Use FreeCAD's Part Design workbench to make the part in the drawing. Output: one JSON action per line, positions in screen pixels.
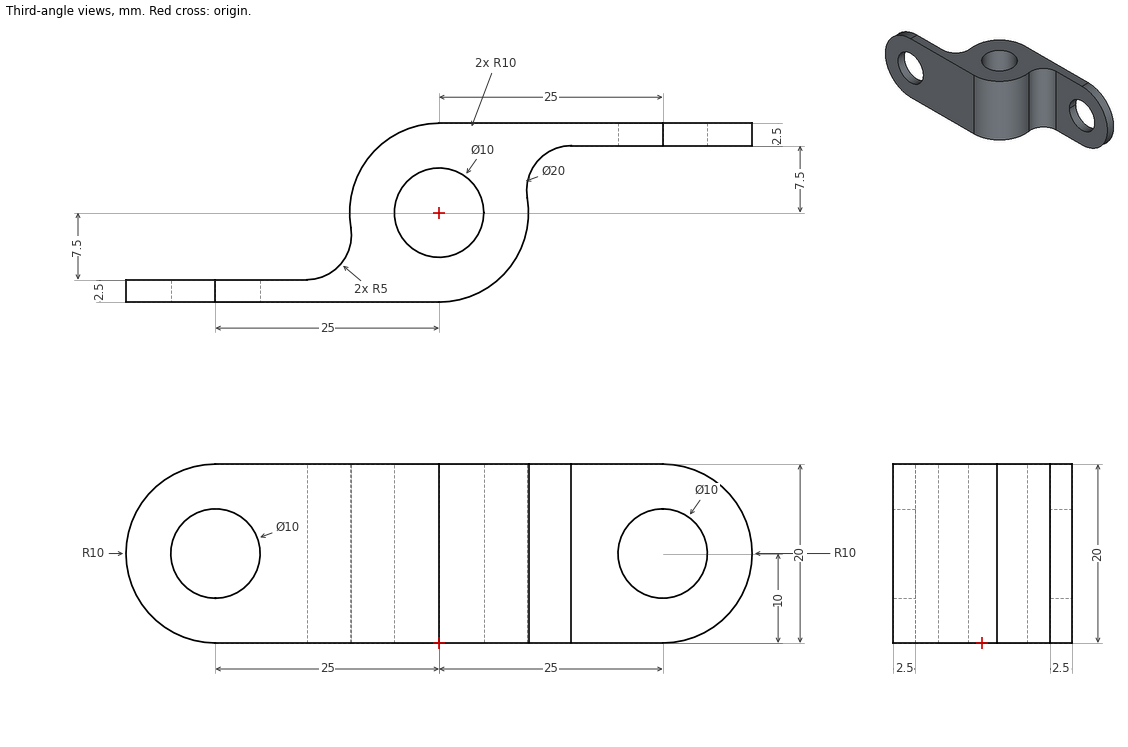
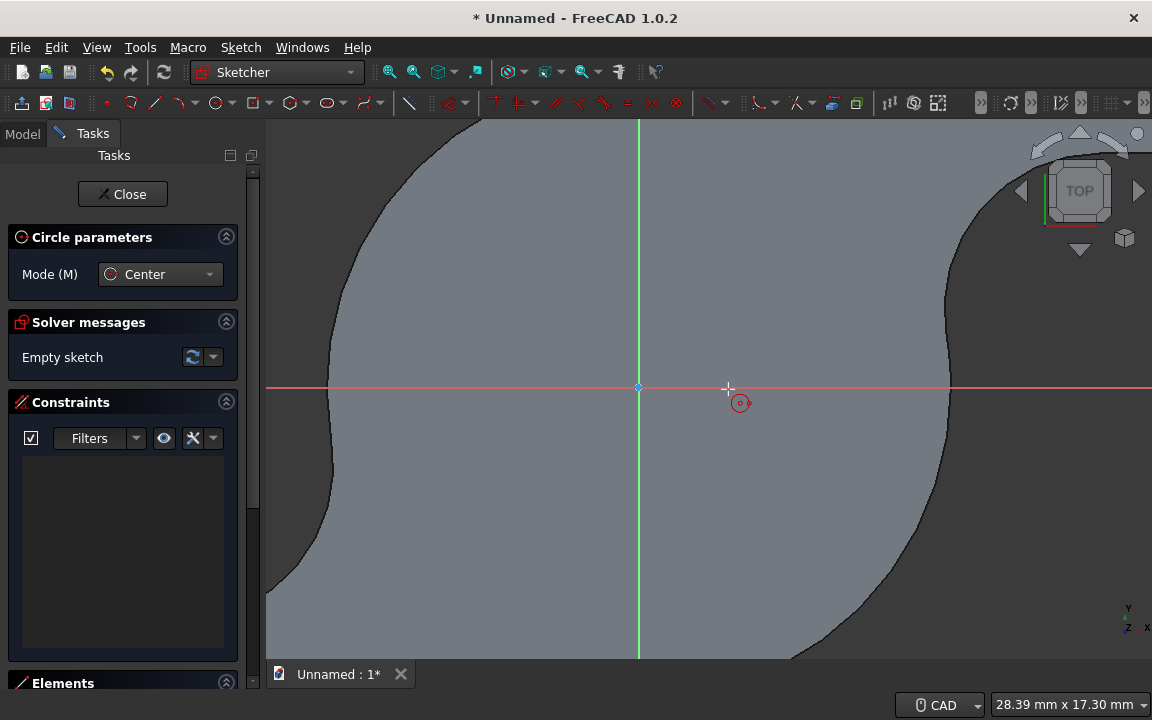
{"action": "left_click", "coordinate": [639, 388]}
{"action": "left_click", "coordinate": [749, 277]}
{"action": "key", "text": "Escape"}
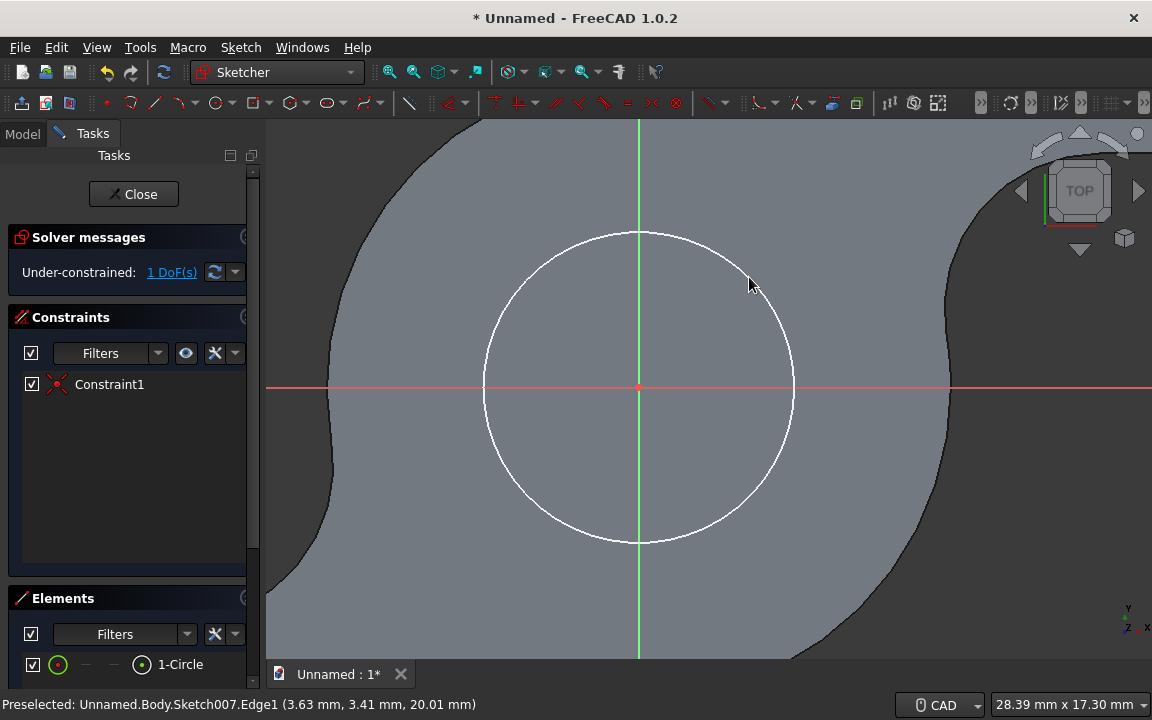
{"action": "left_click", "coordinate": [448, 104]}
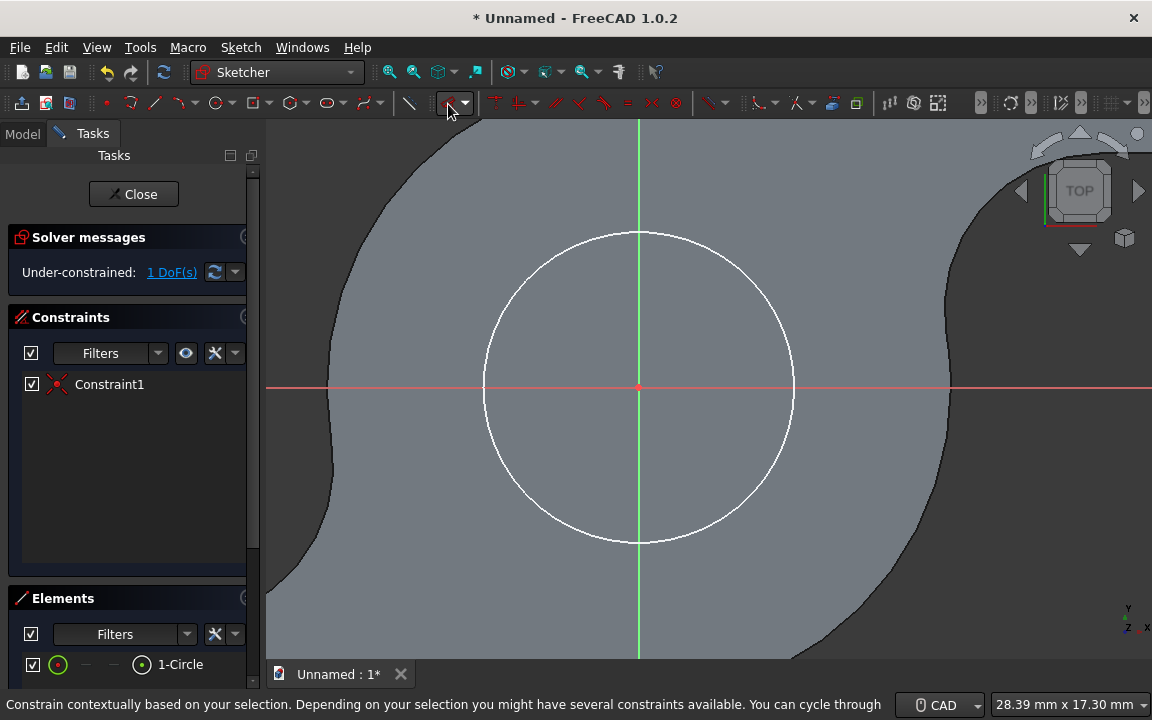
{"action": "left_click", "coordinate": [748, 277]}
{"action": "left_click", "coordinate": [770, 254]}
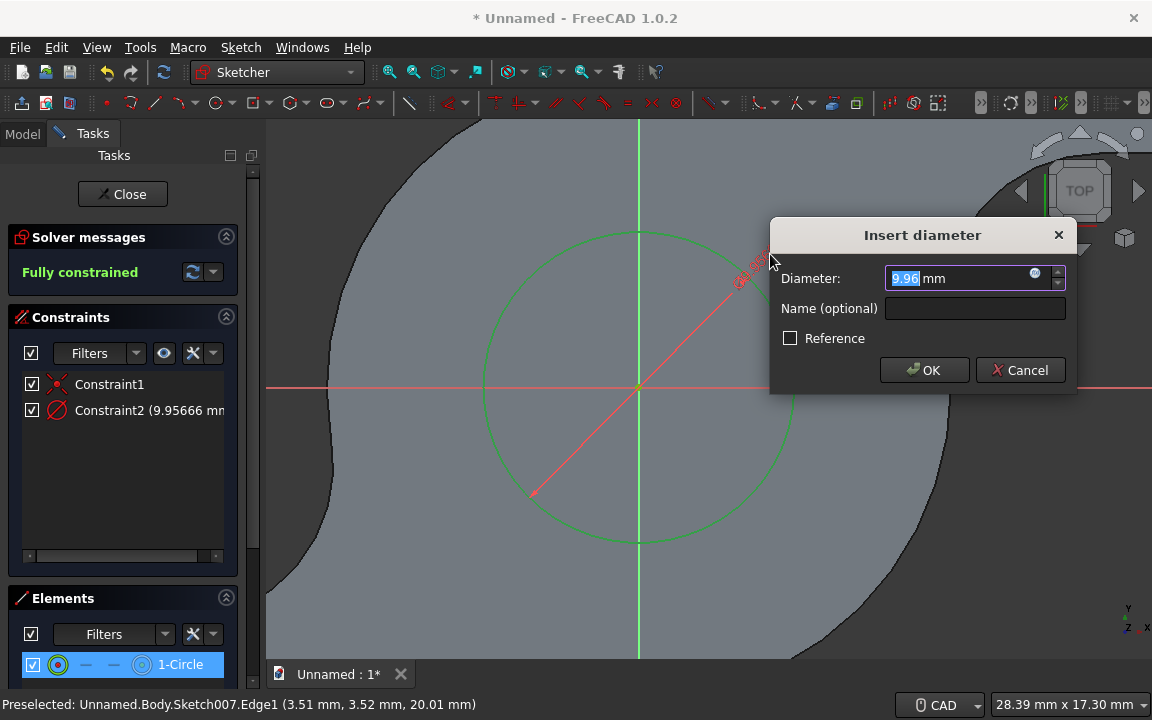
{"action": "type", "text": "10"}
{"action": "key", "text": "Return"}
{"action": "key", "text": "Escape"}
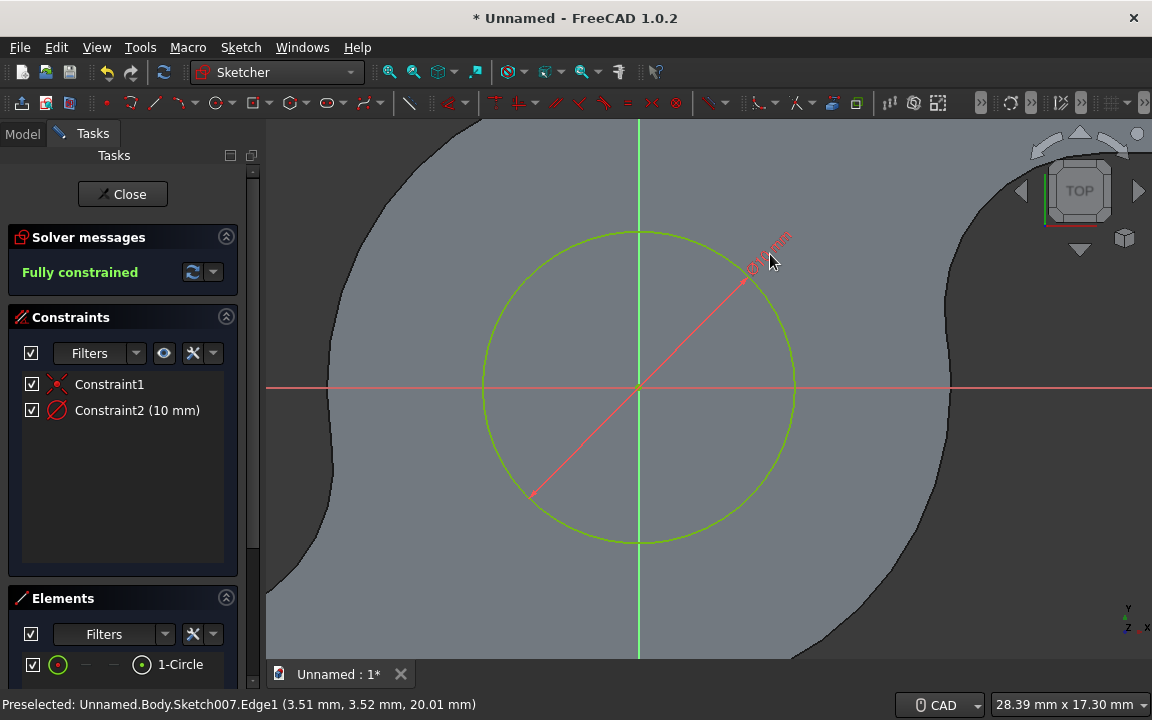
{"action": "left_click", "coordinate": [123, 194]}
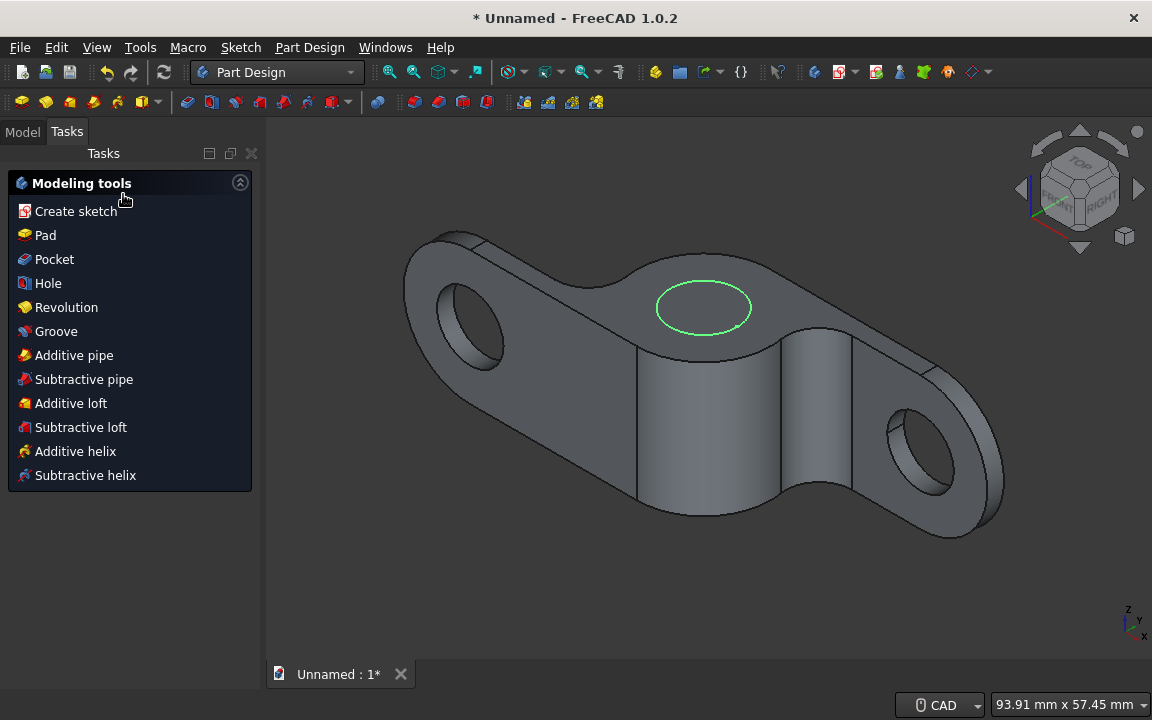
{"action": "left_click", "coordinate": [188, 102]}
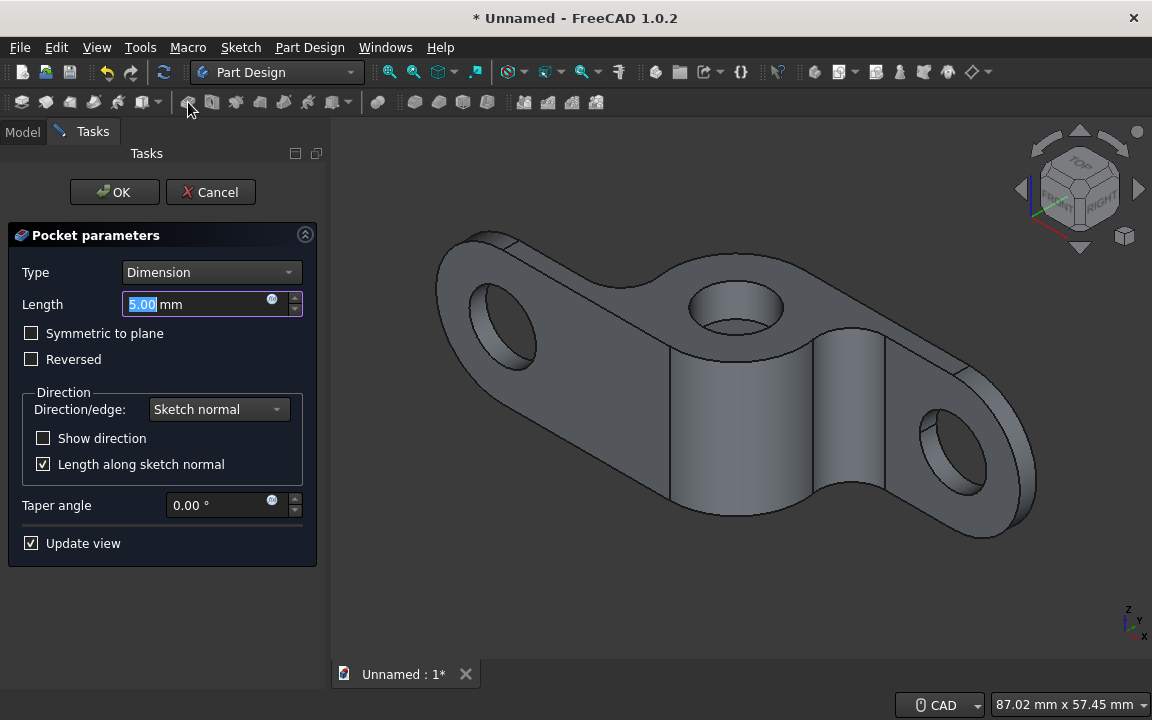
{"action": "type", "text": "20"}
{"action": "key", "text": "Tab"}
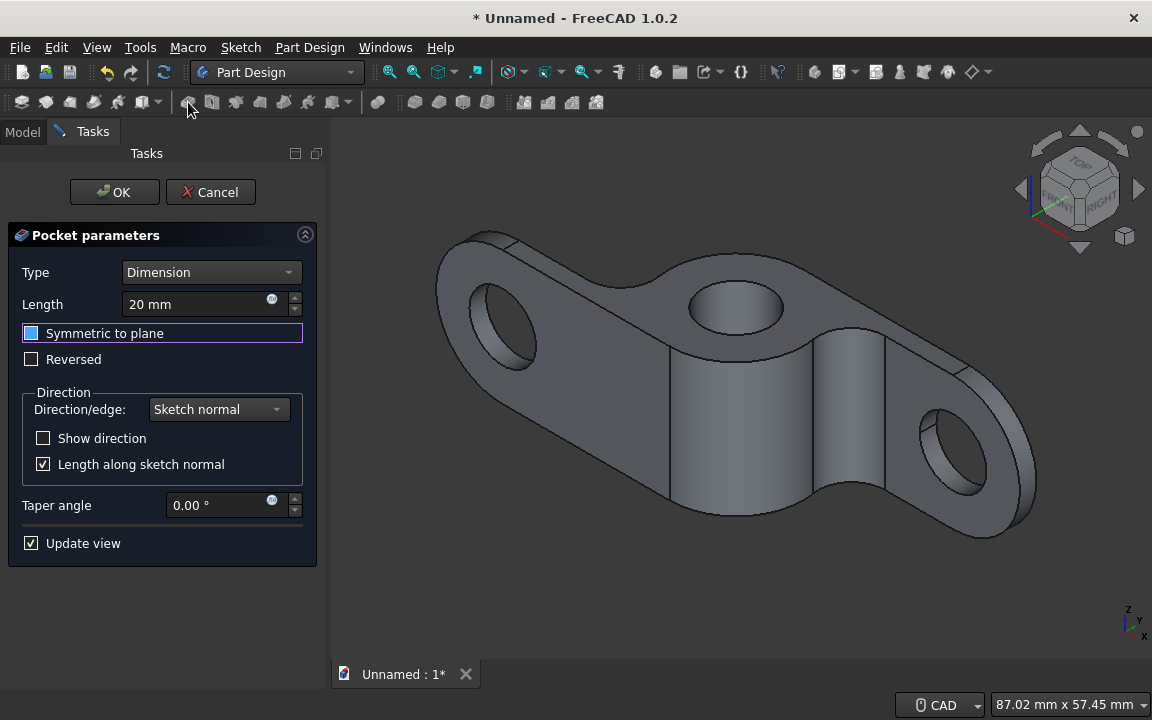
{"action": "left_click", "coordinate": [115, 192]}